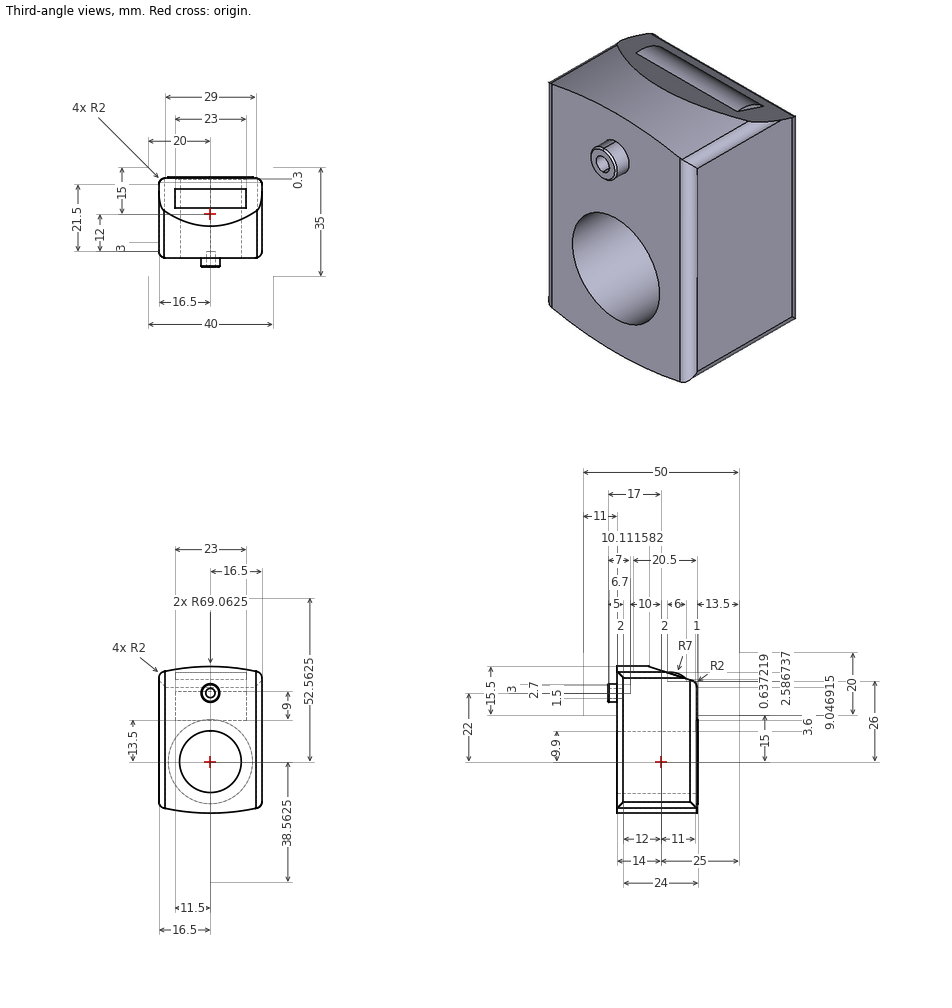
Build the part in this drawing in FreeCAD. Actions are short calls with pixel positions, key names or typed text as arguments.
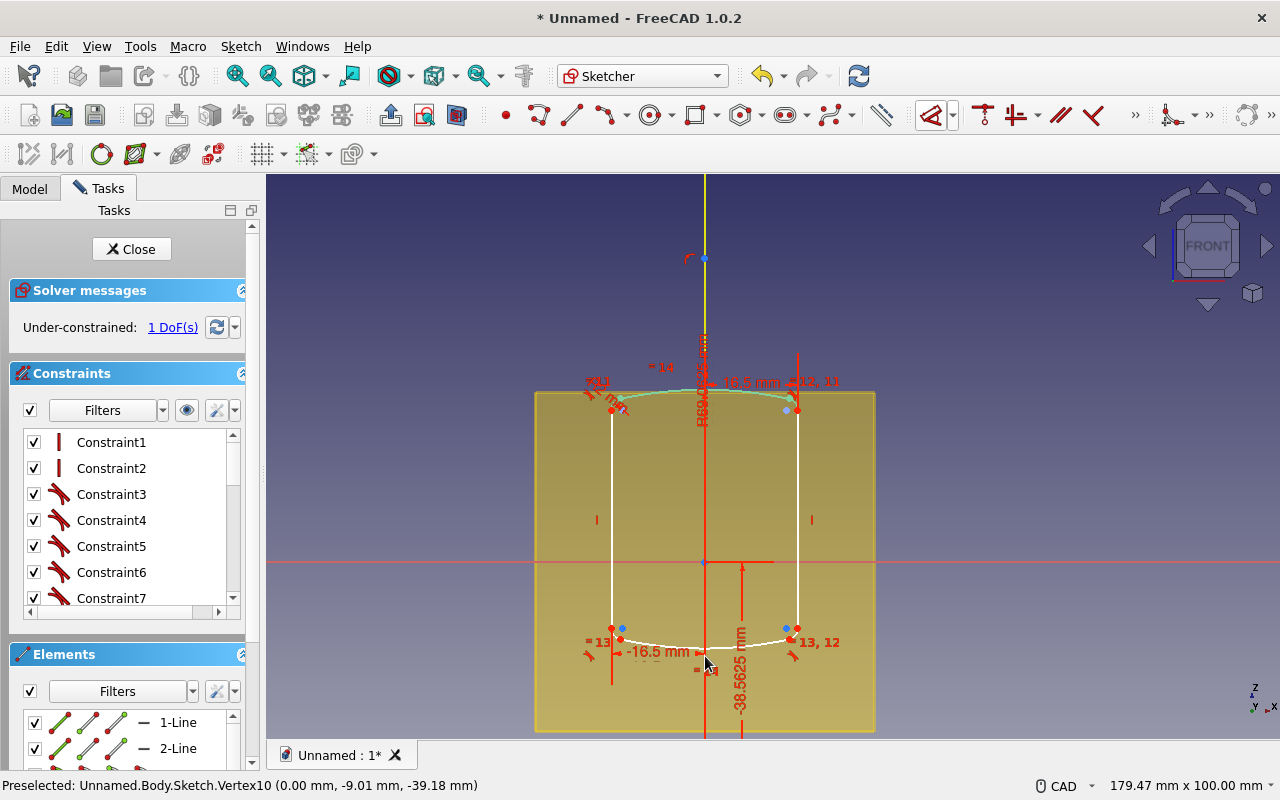
click(705, 258)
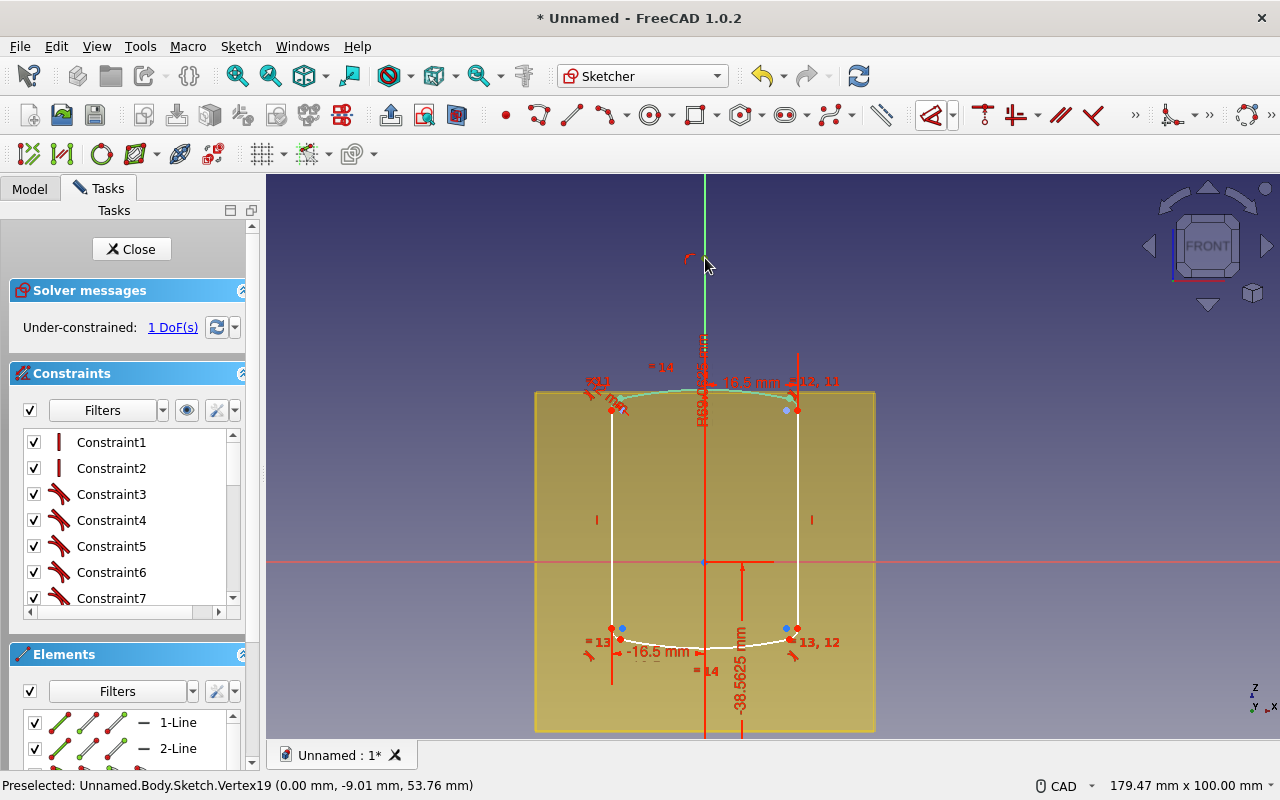
click(952, 116)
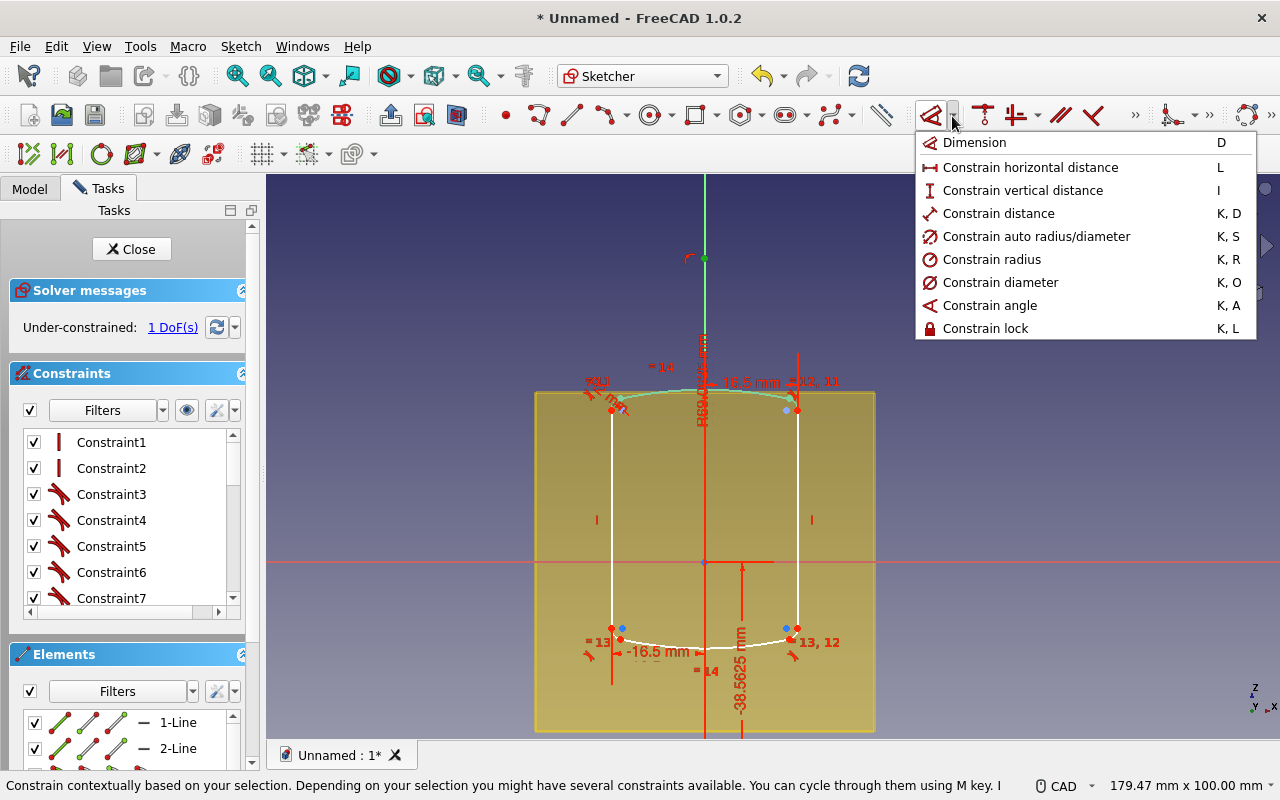
click(1086, 190)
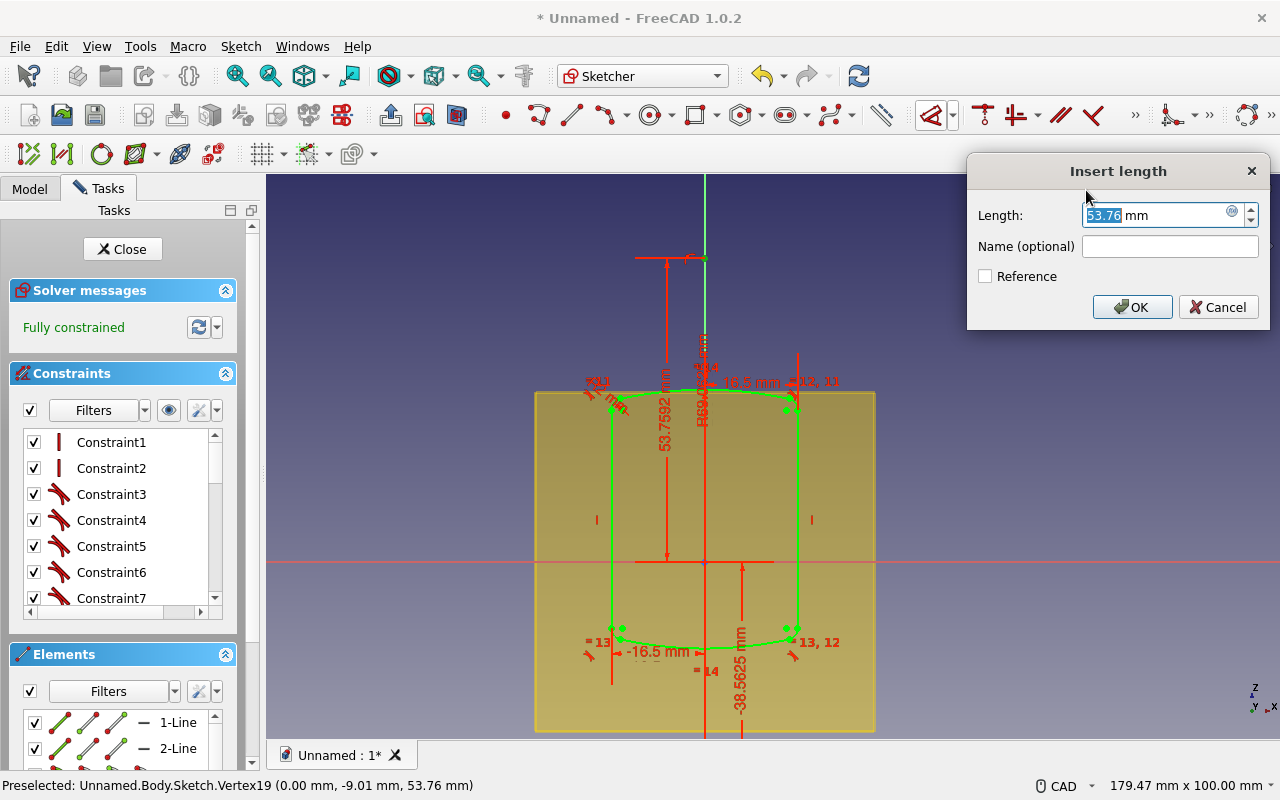
text(52.5625)
key(Return)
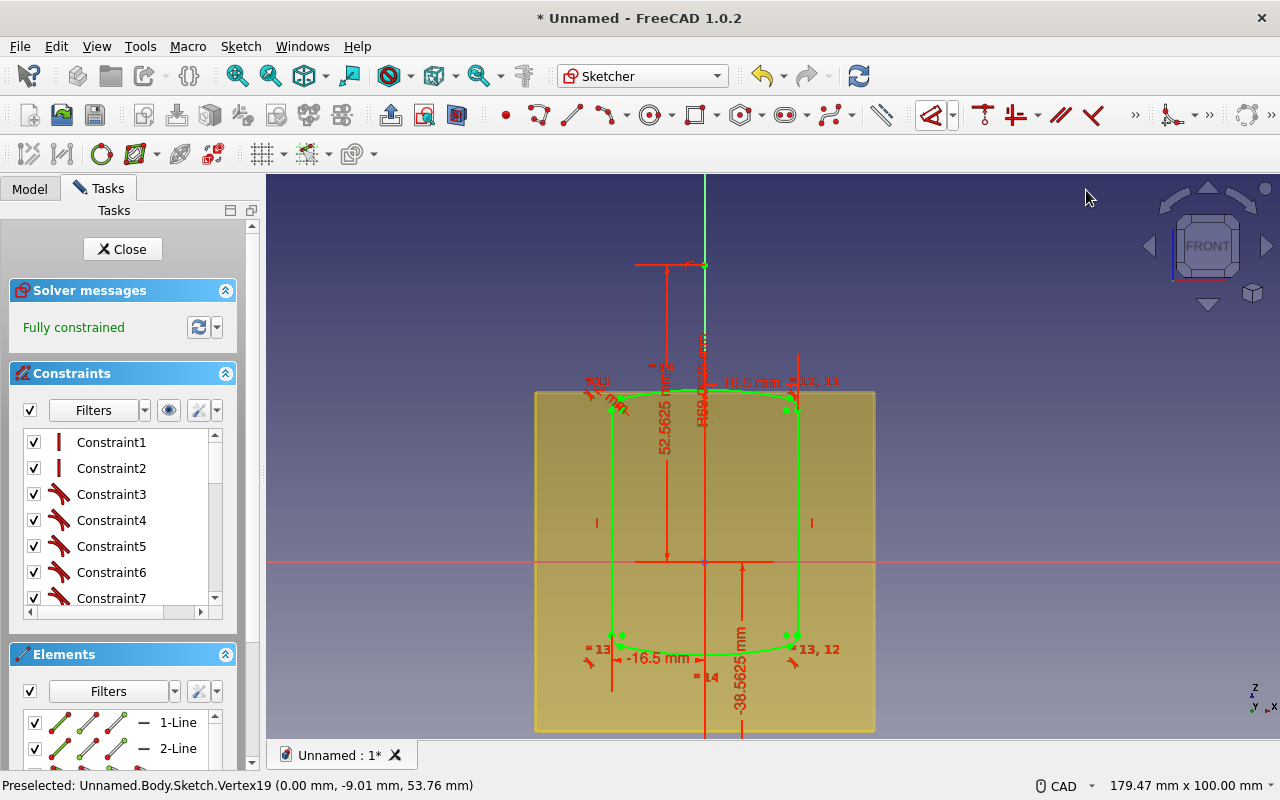
click(123, 249)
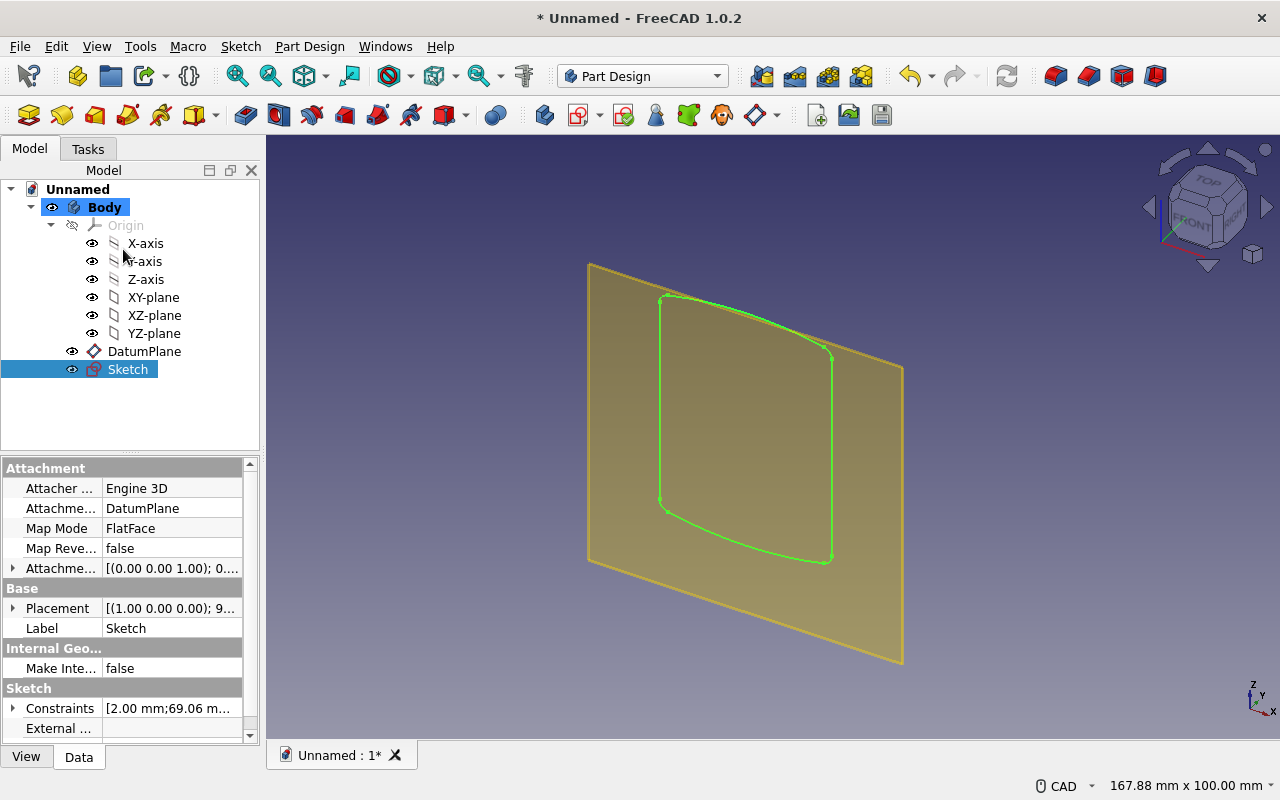
click(29, 116)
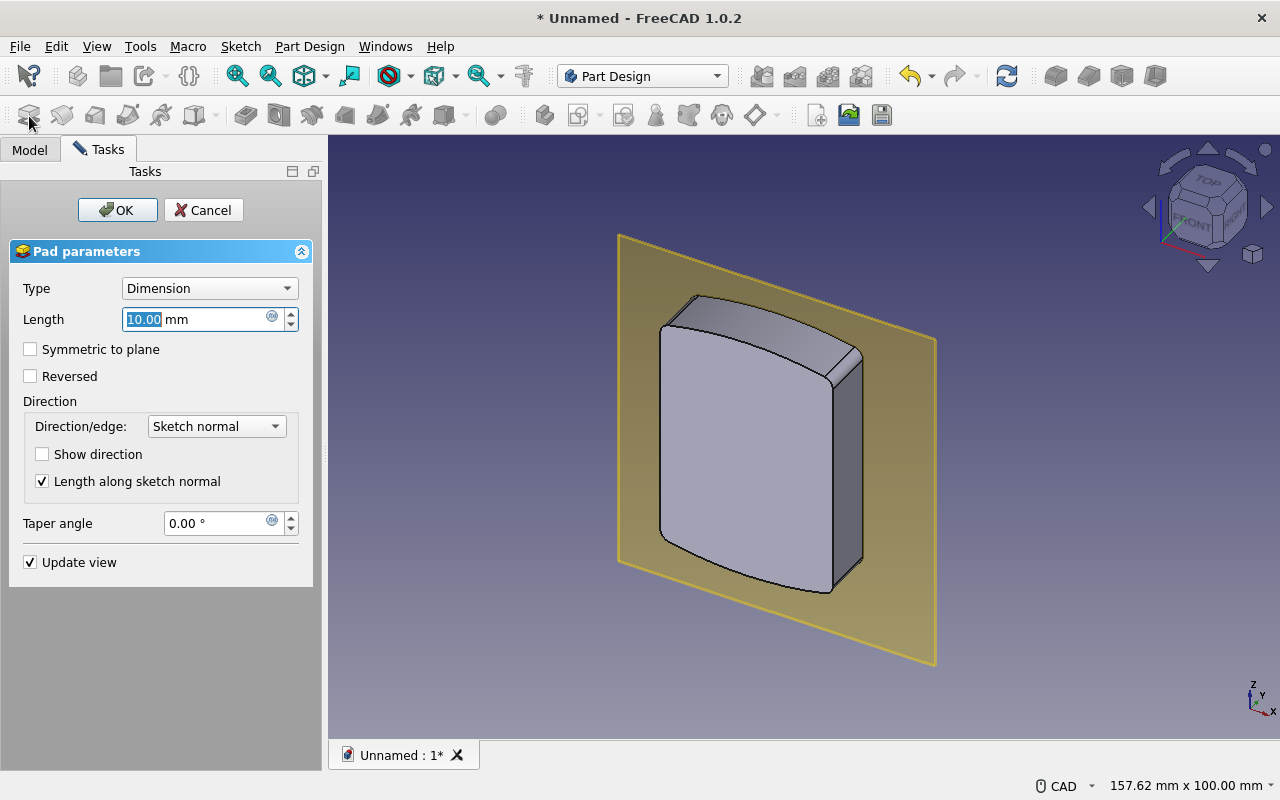
text(20.5)
key(Tab)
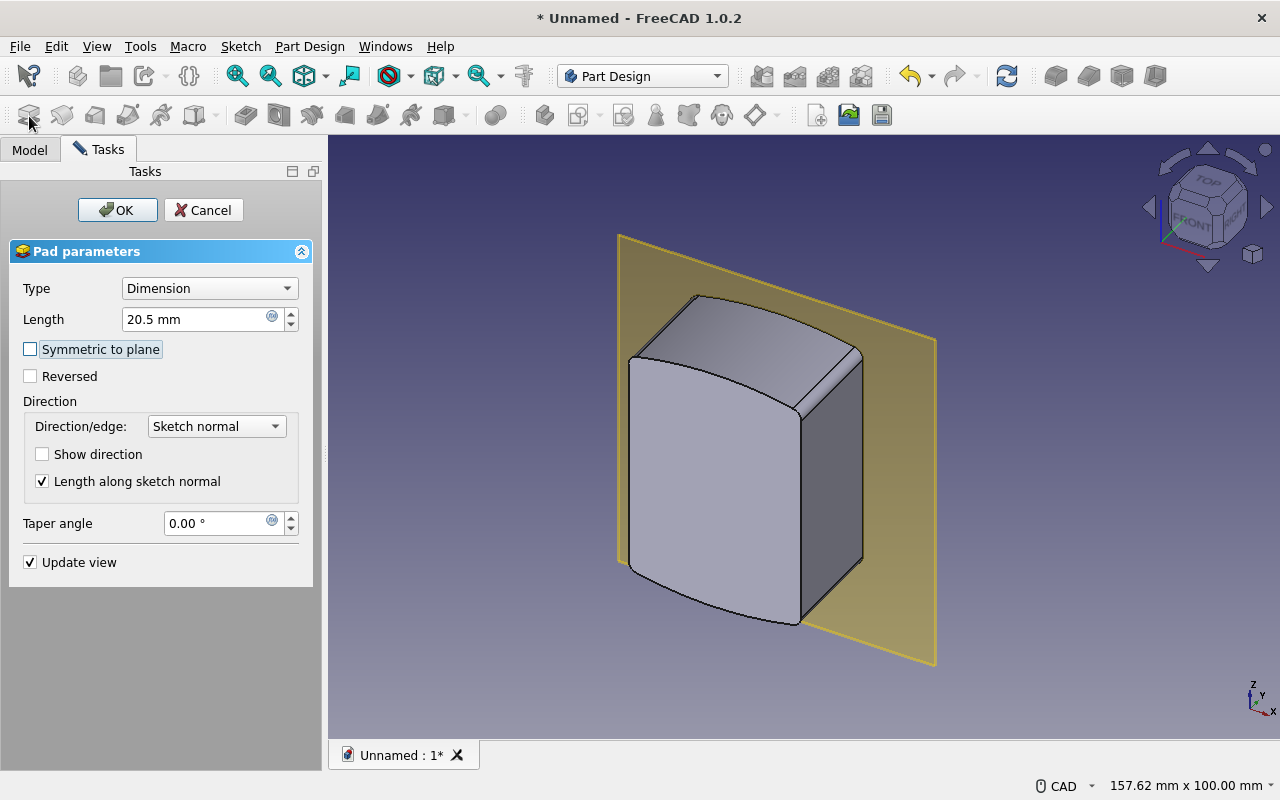
click(31, 376)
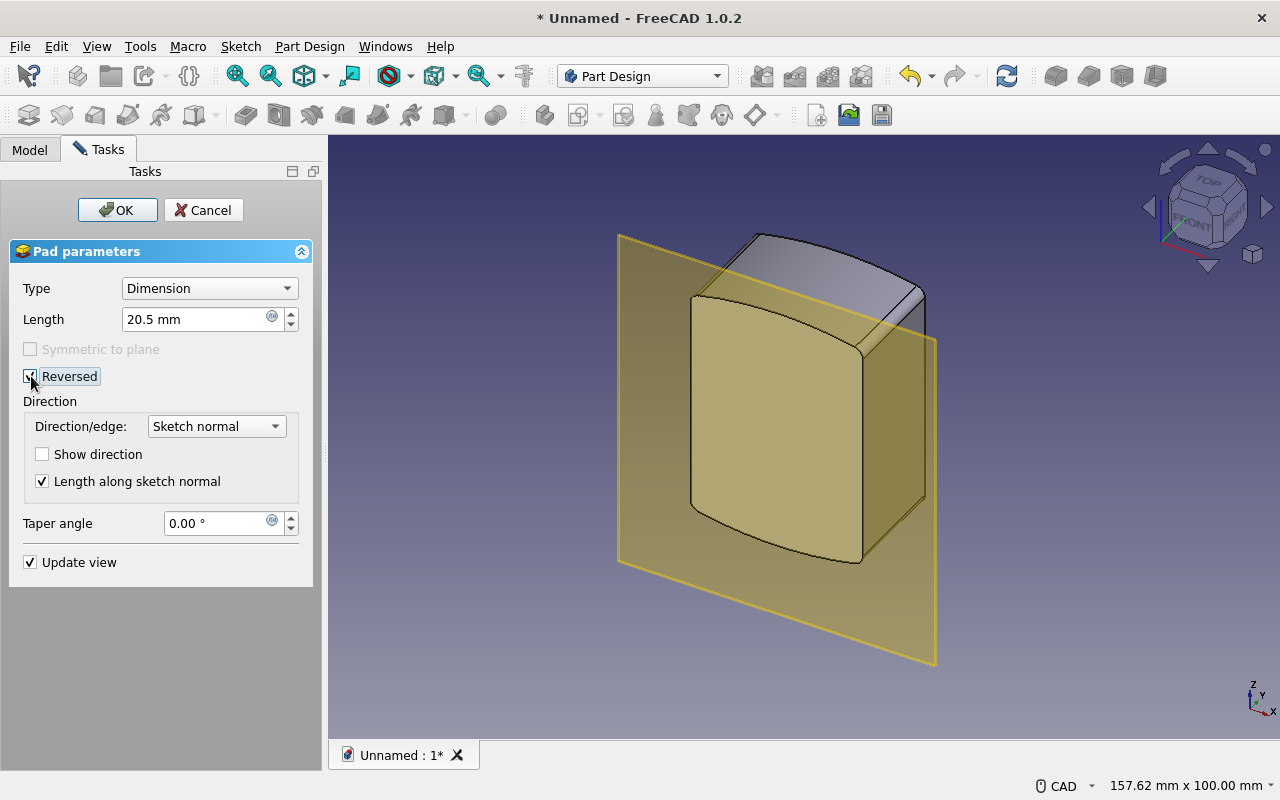
click(118, 210)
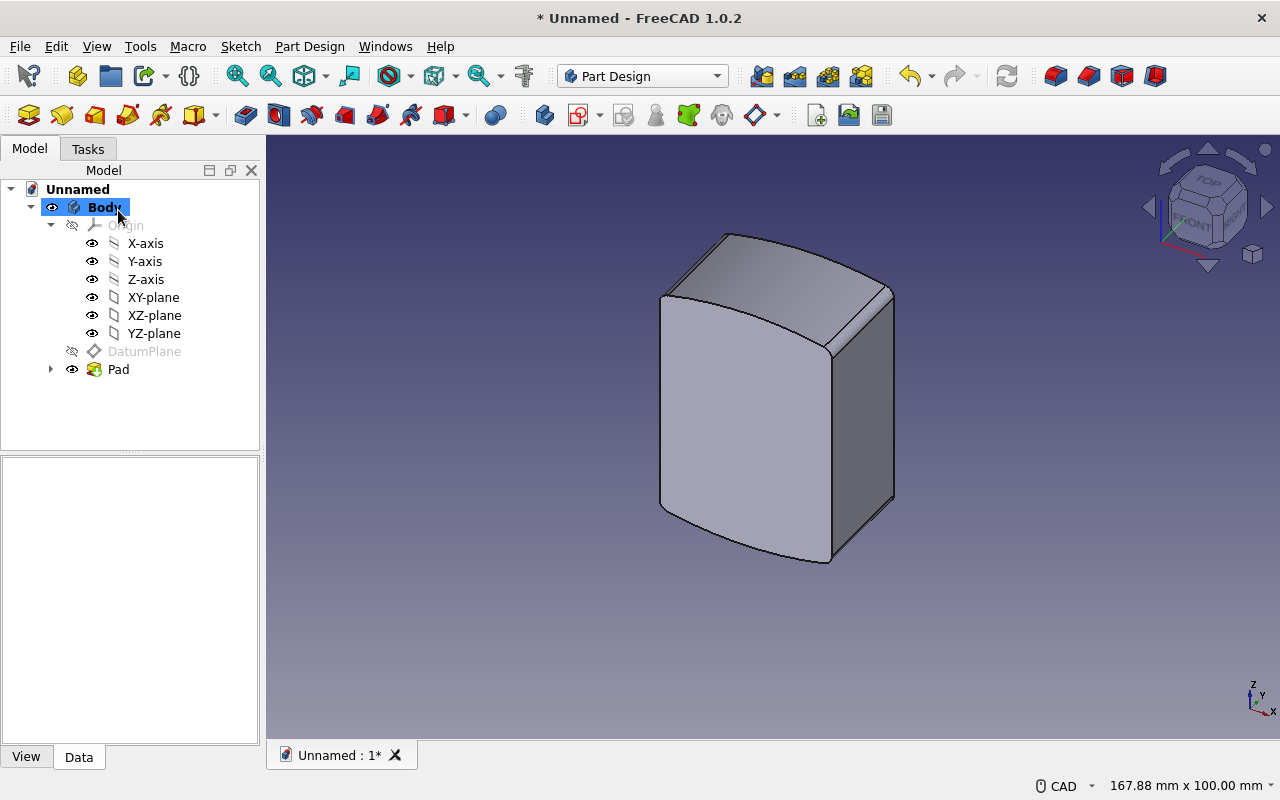
click(137, 315)